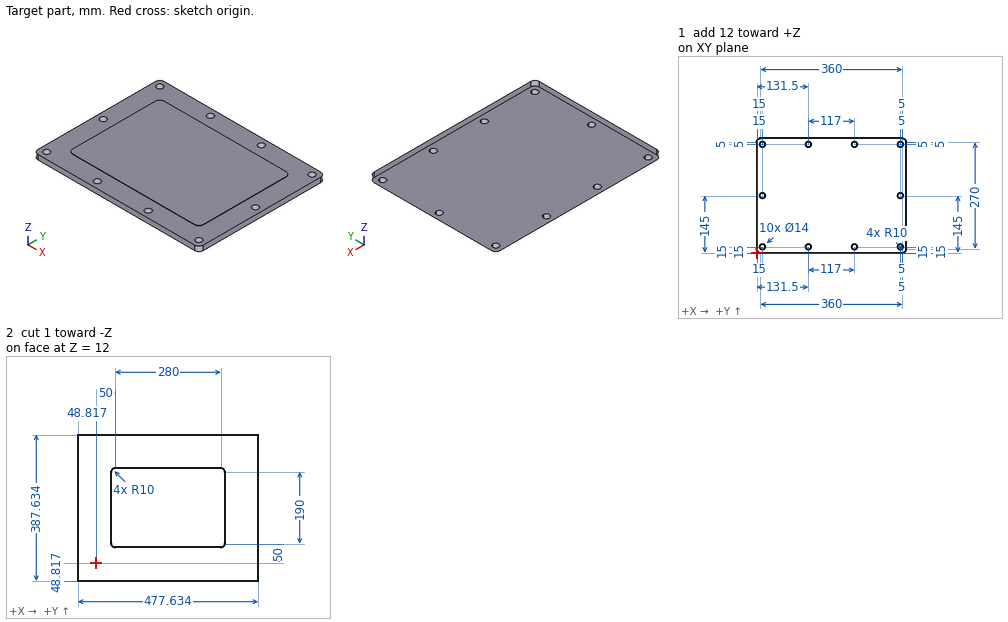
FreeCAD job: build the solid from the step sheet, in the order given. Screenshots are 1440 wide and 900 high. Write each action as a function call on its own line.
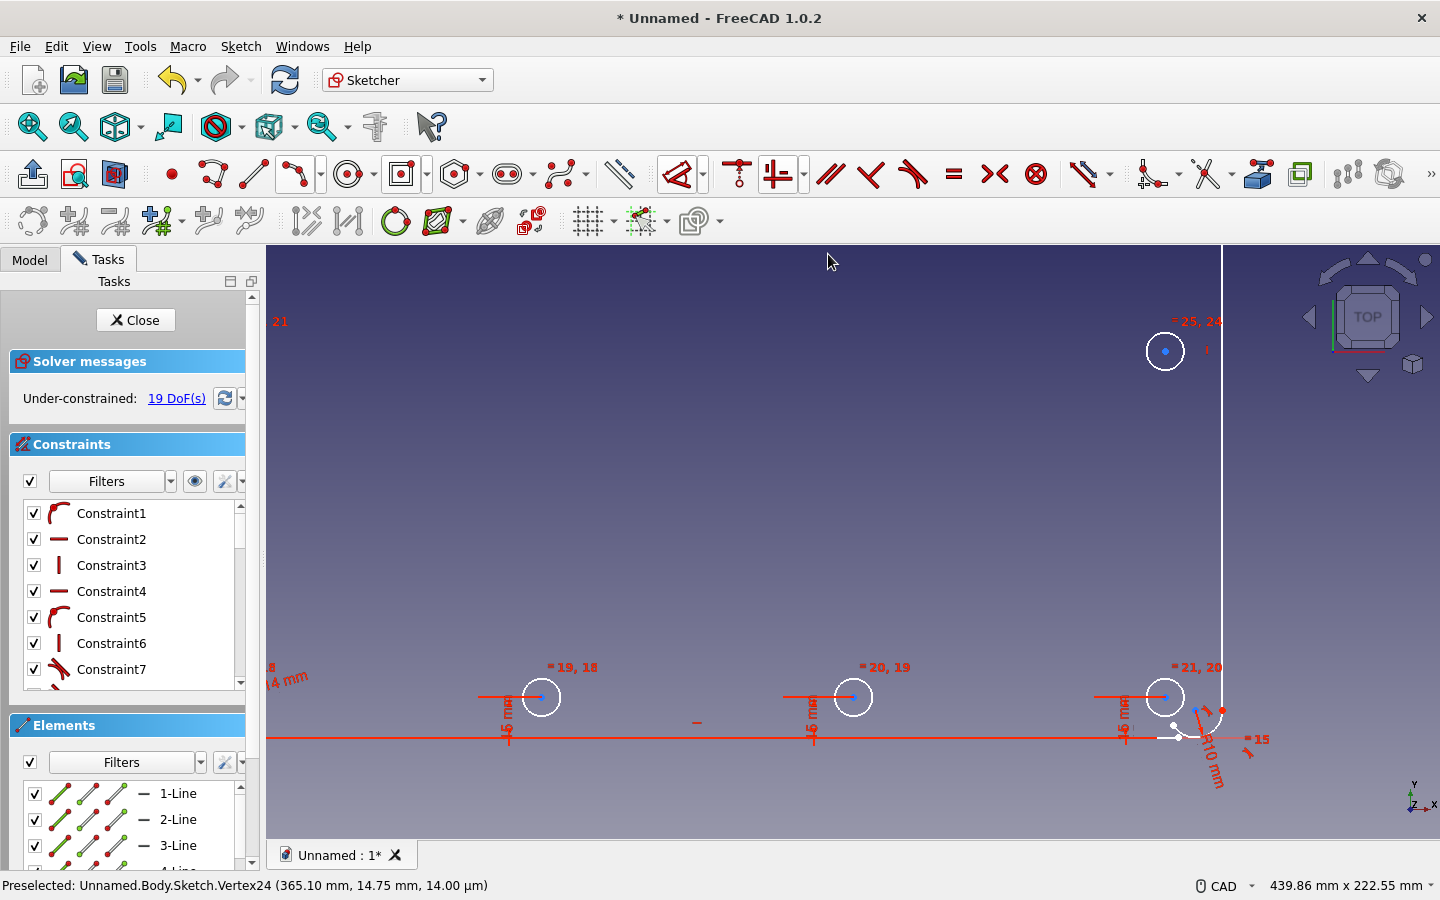
scroll(855, 698, down, 4)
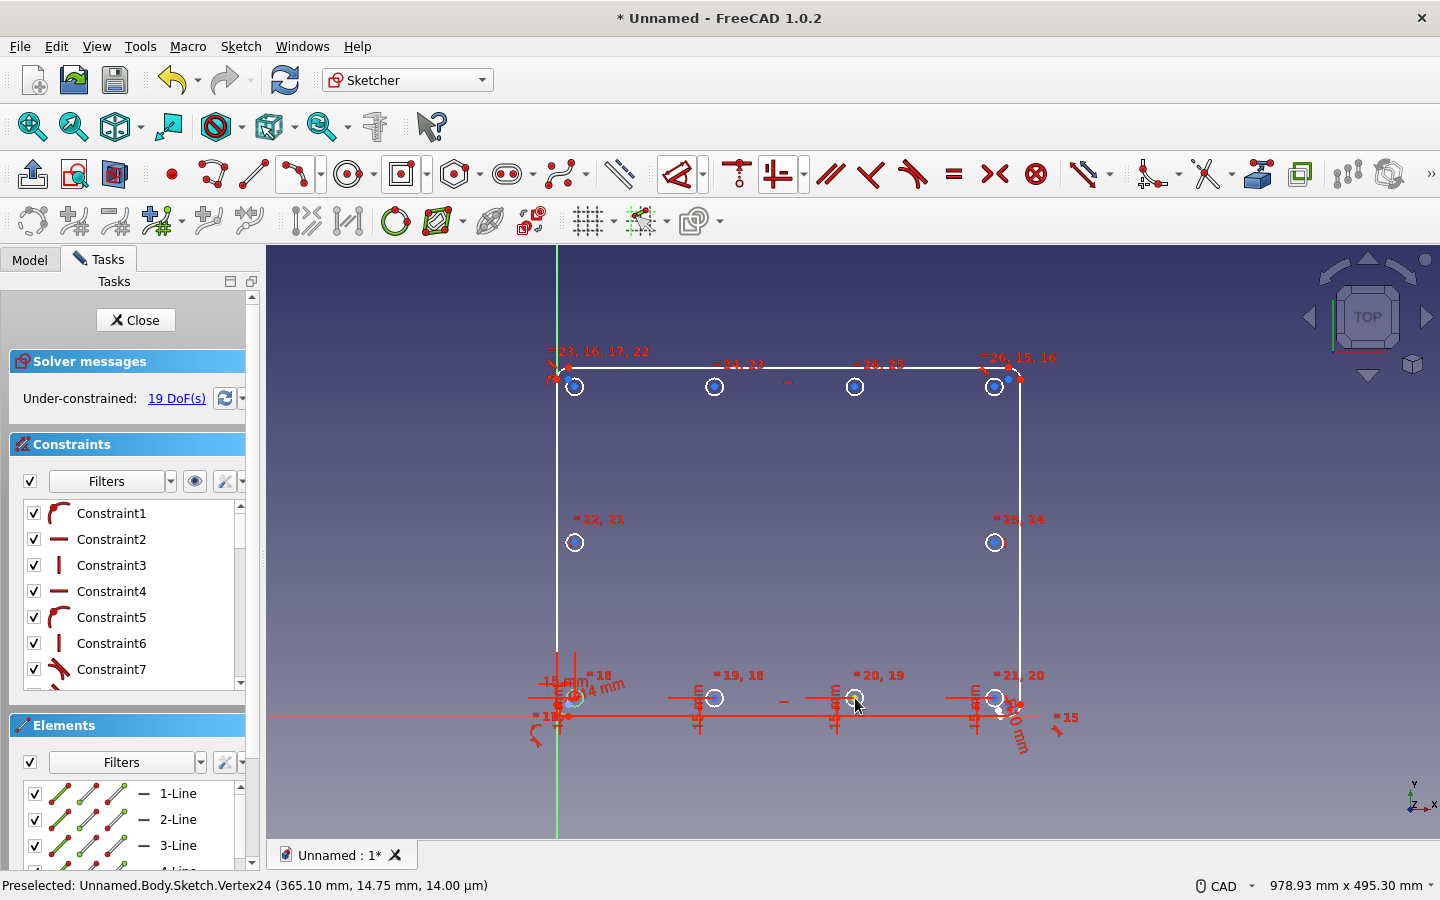
scroll(575, 543, up, 4)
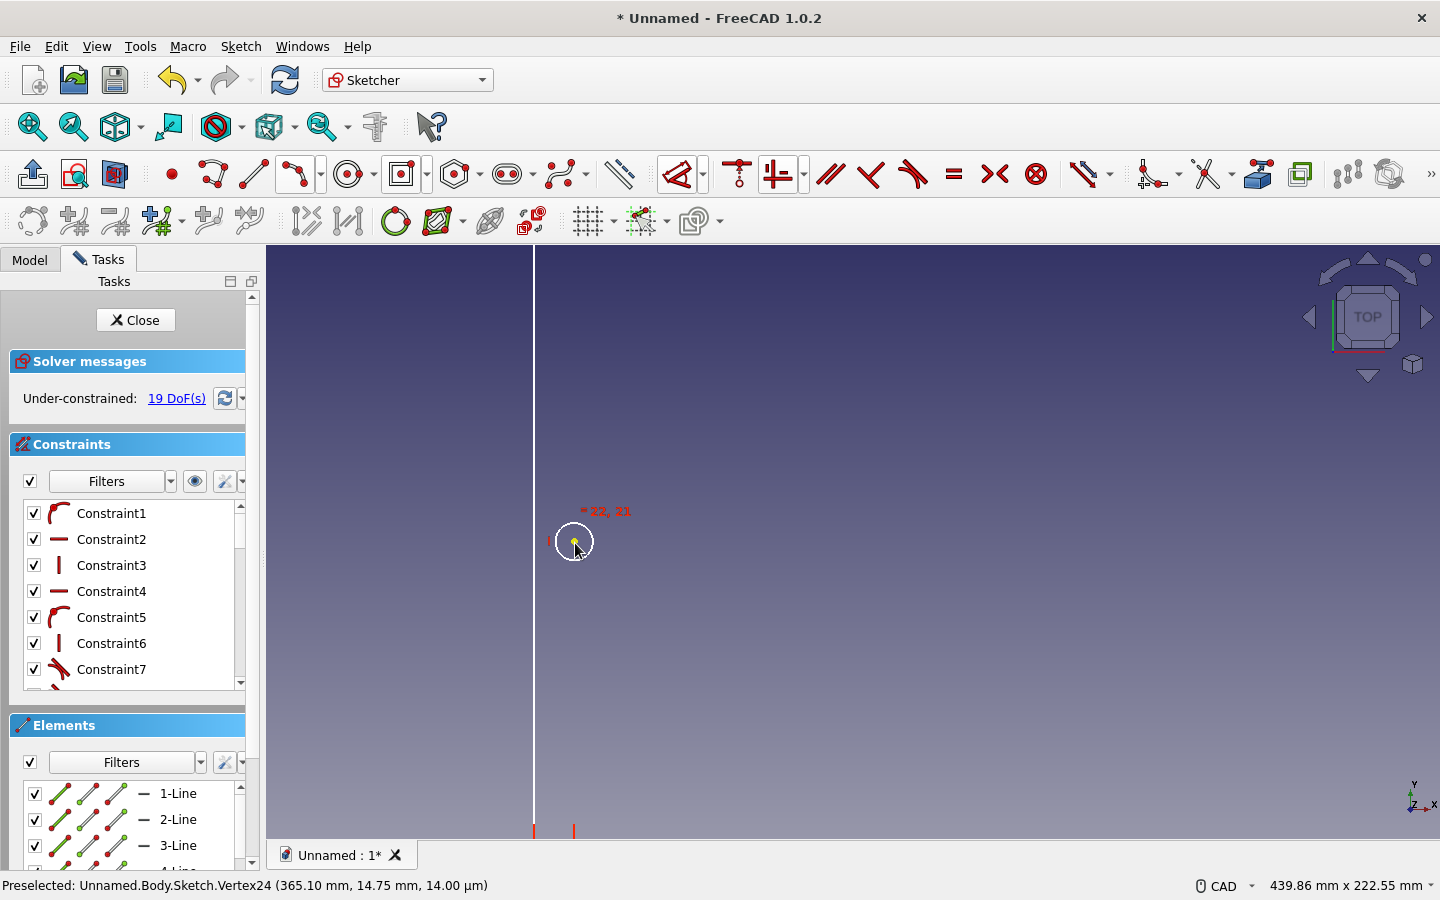
click(574, 542)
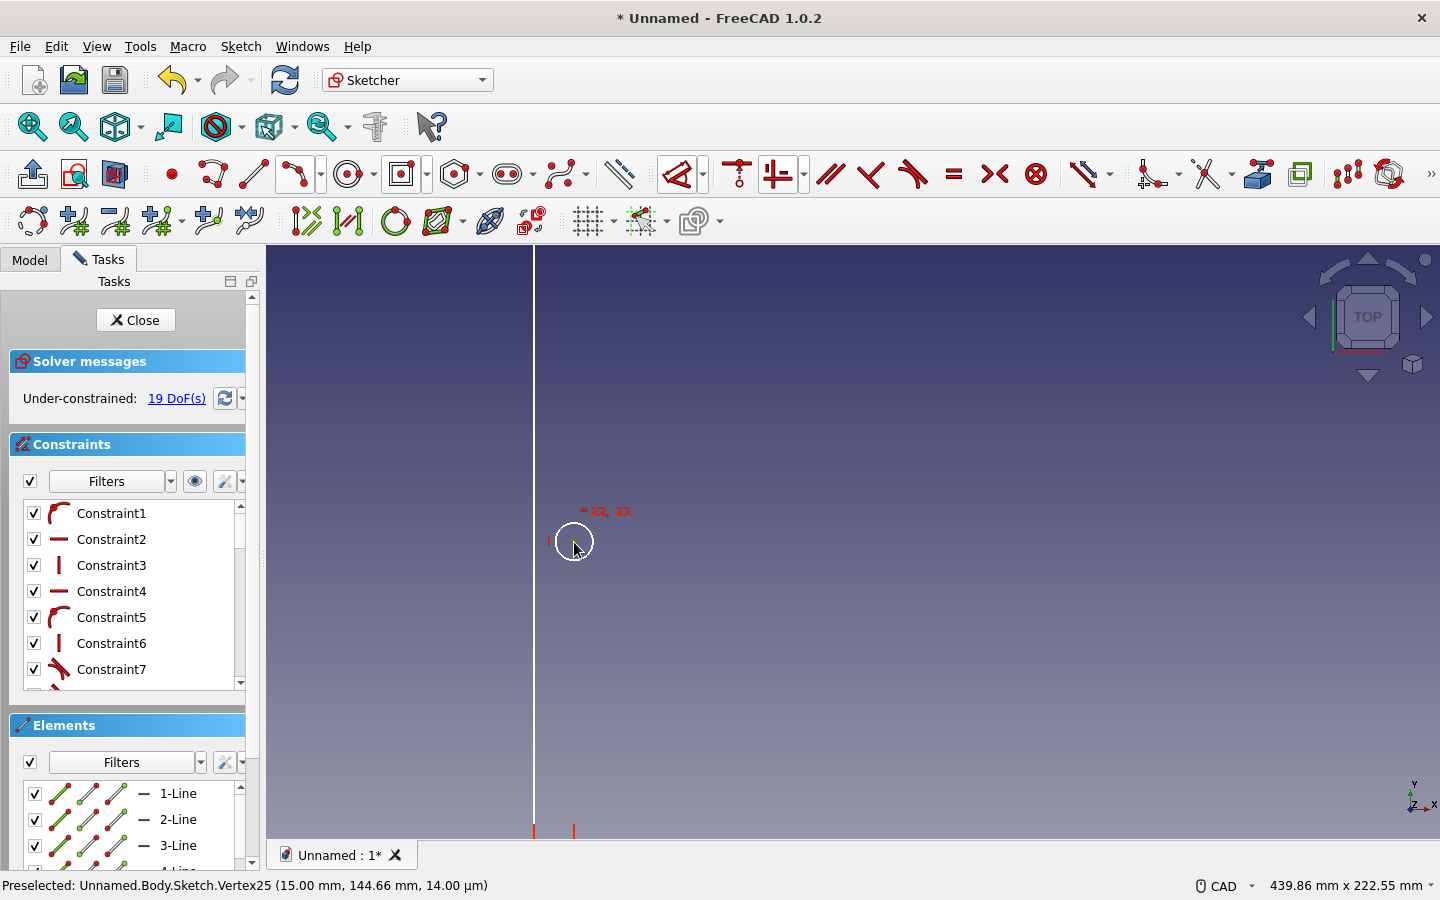
key(l)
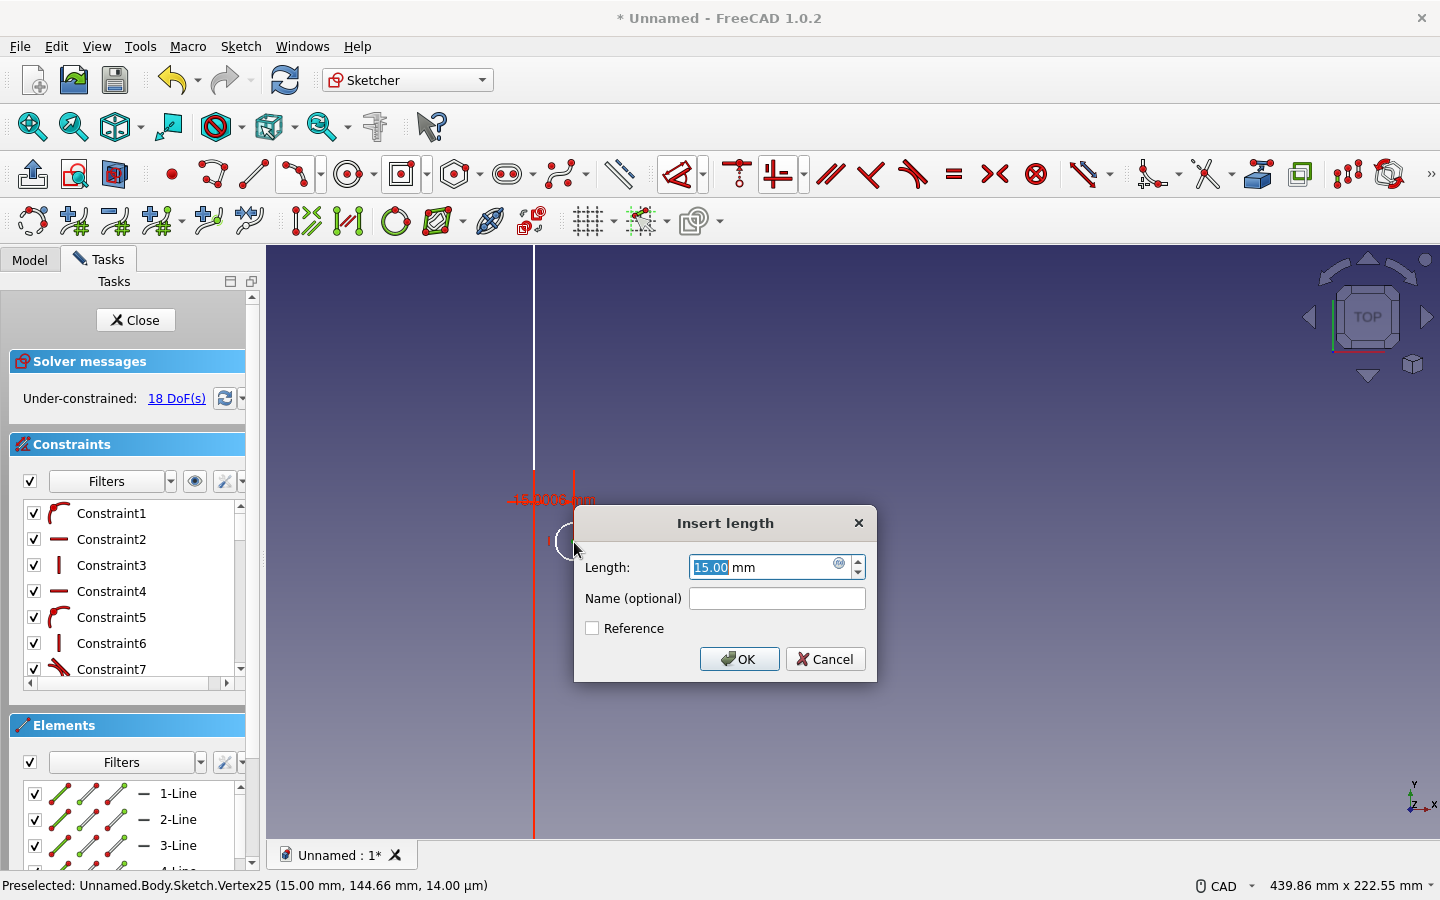
text(15)
key(Return)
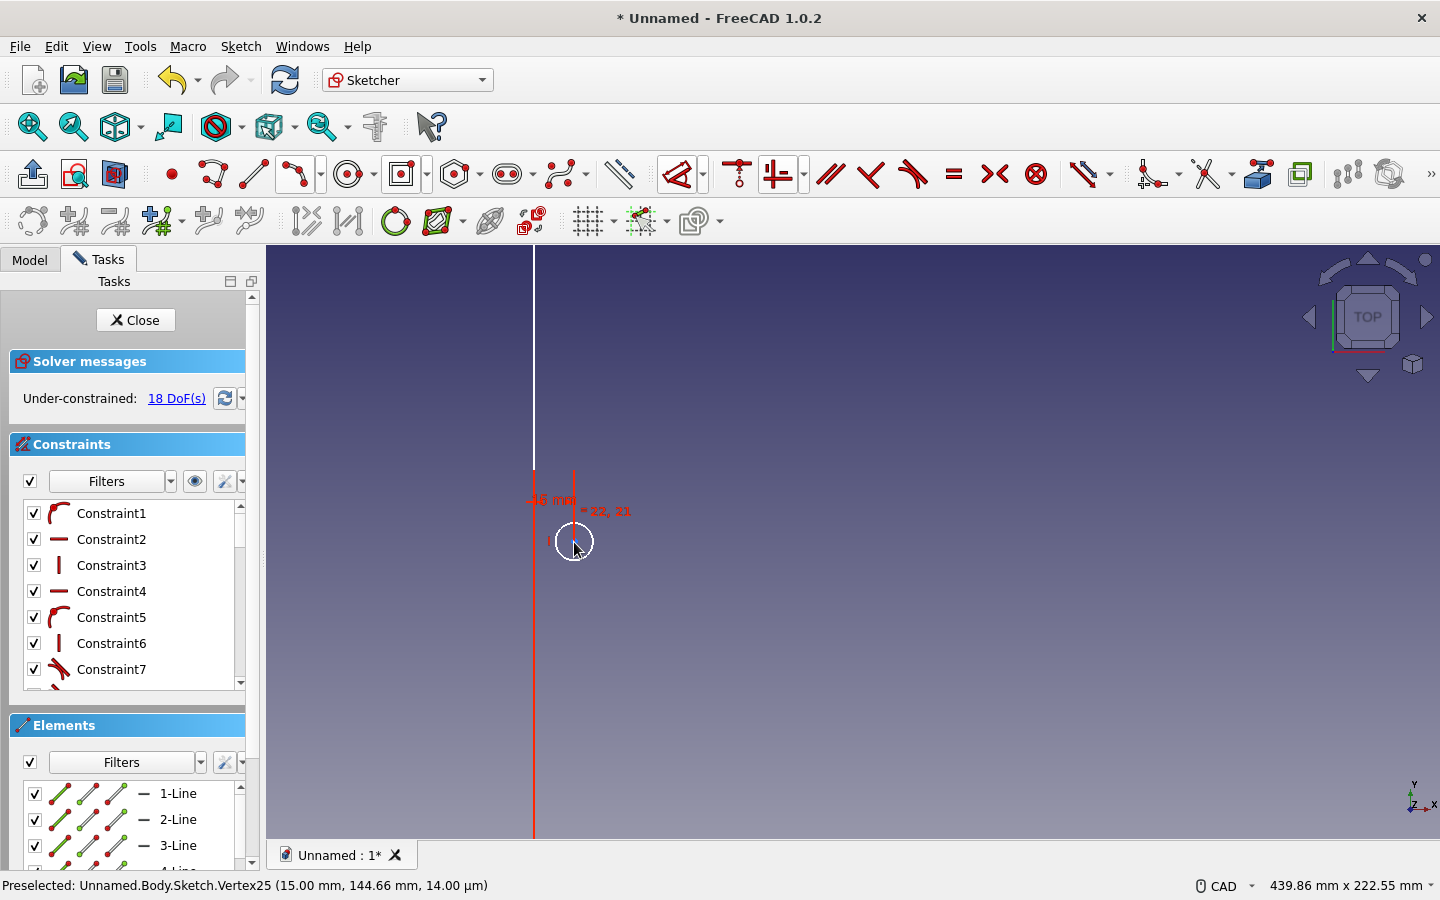
scroll(575, 543, down, 4)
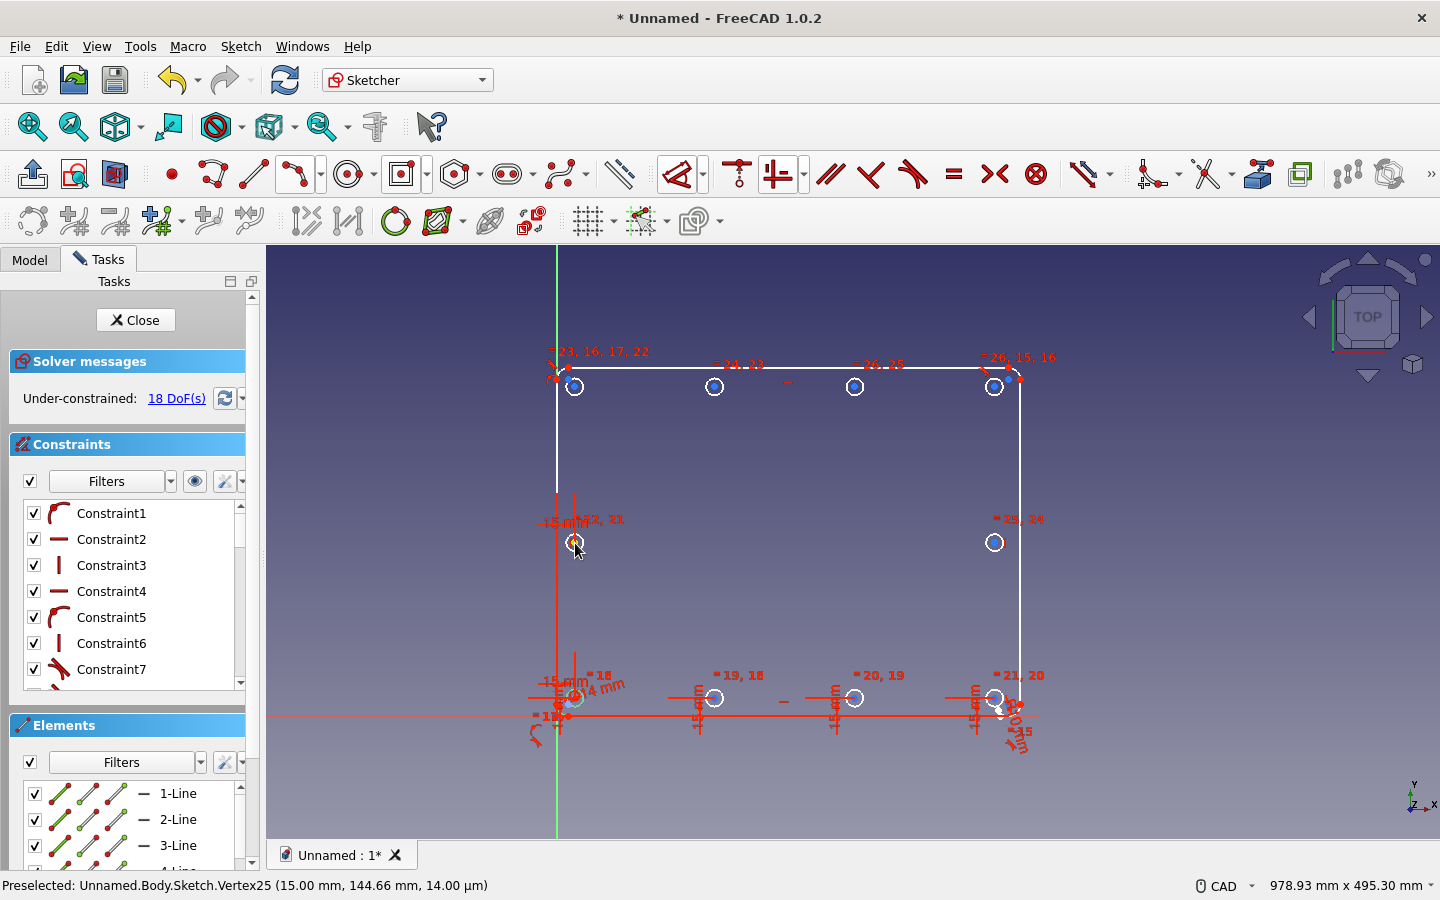
scroll(575, 387, up, 4)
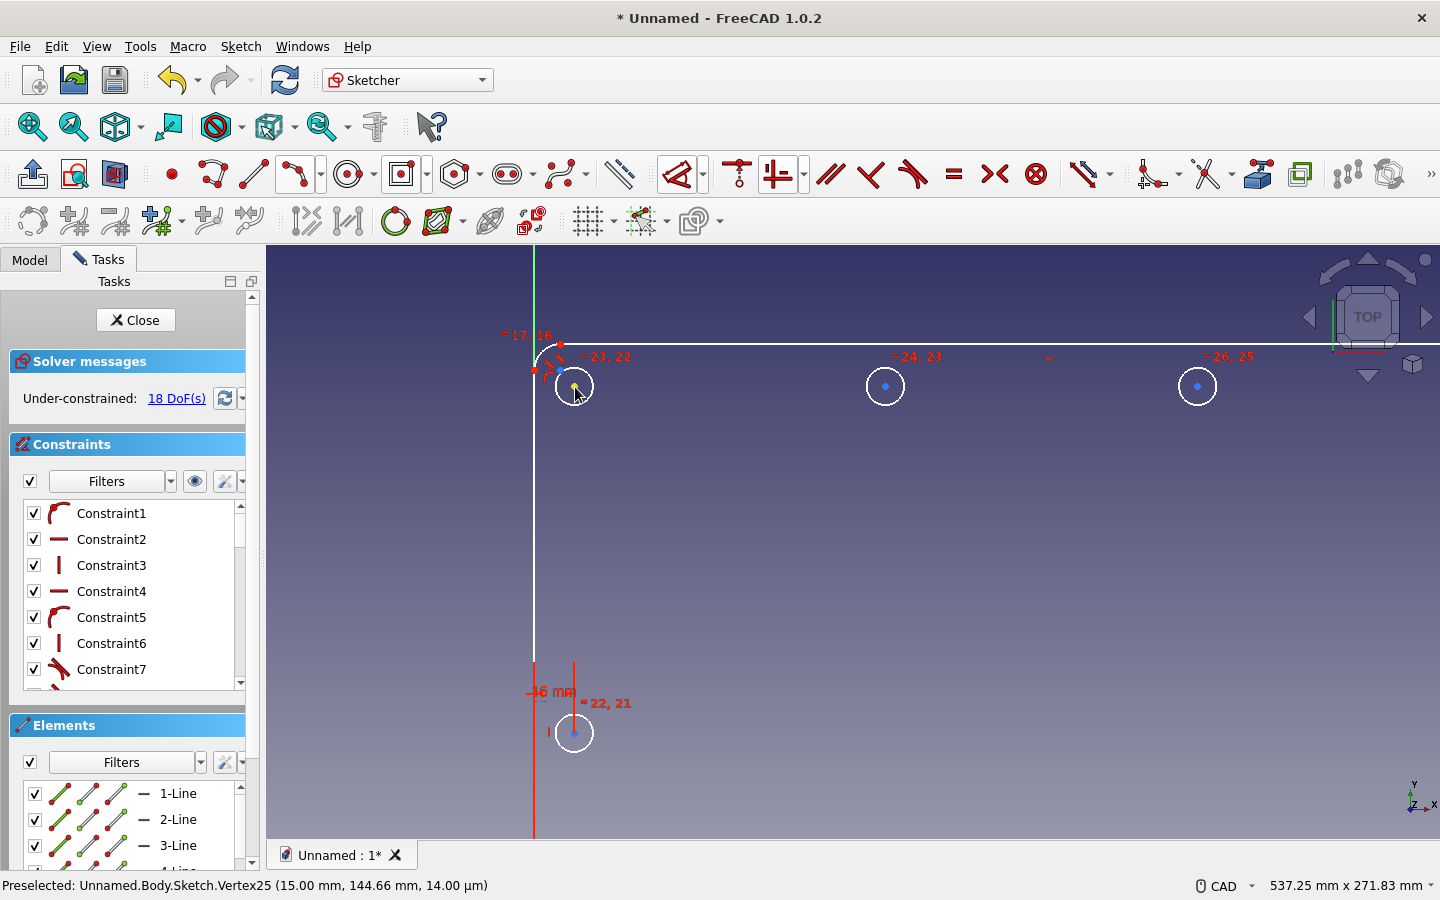
click(574, 386)